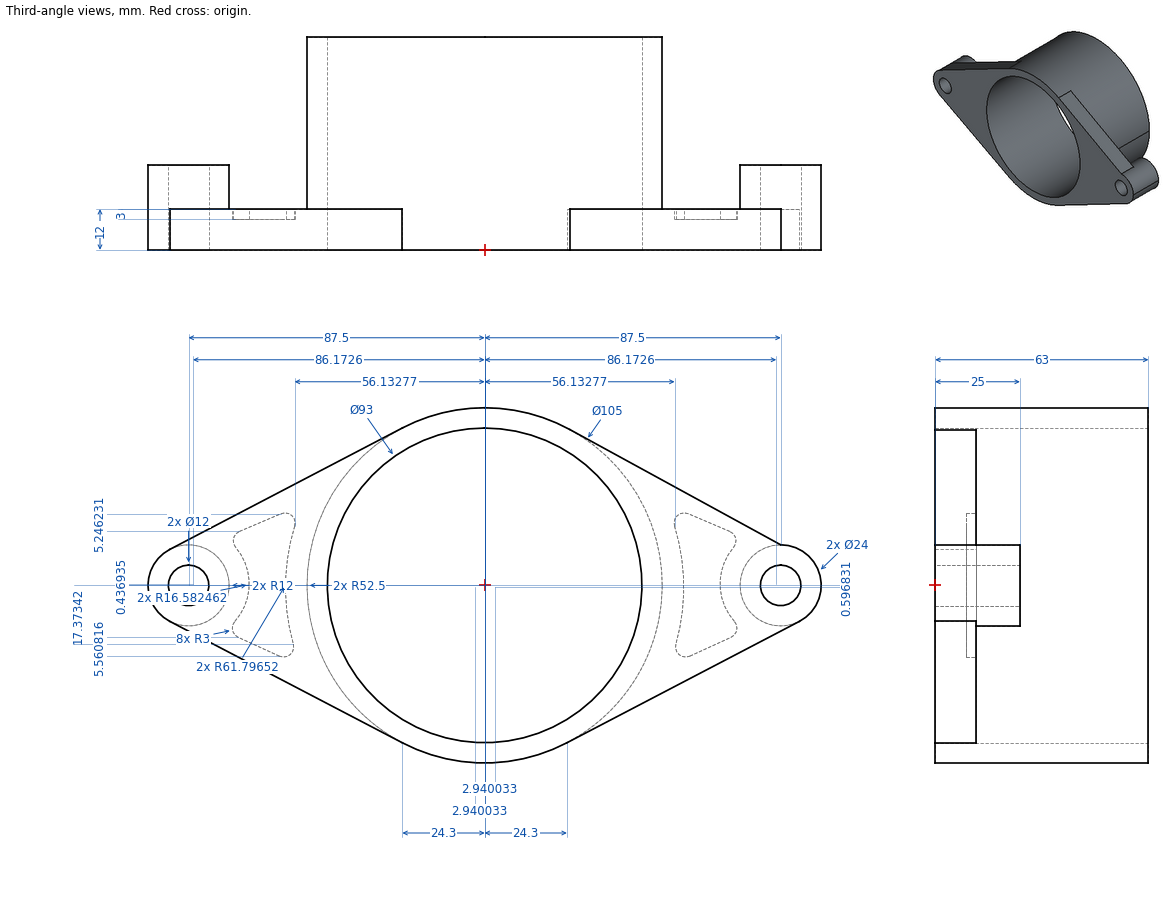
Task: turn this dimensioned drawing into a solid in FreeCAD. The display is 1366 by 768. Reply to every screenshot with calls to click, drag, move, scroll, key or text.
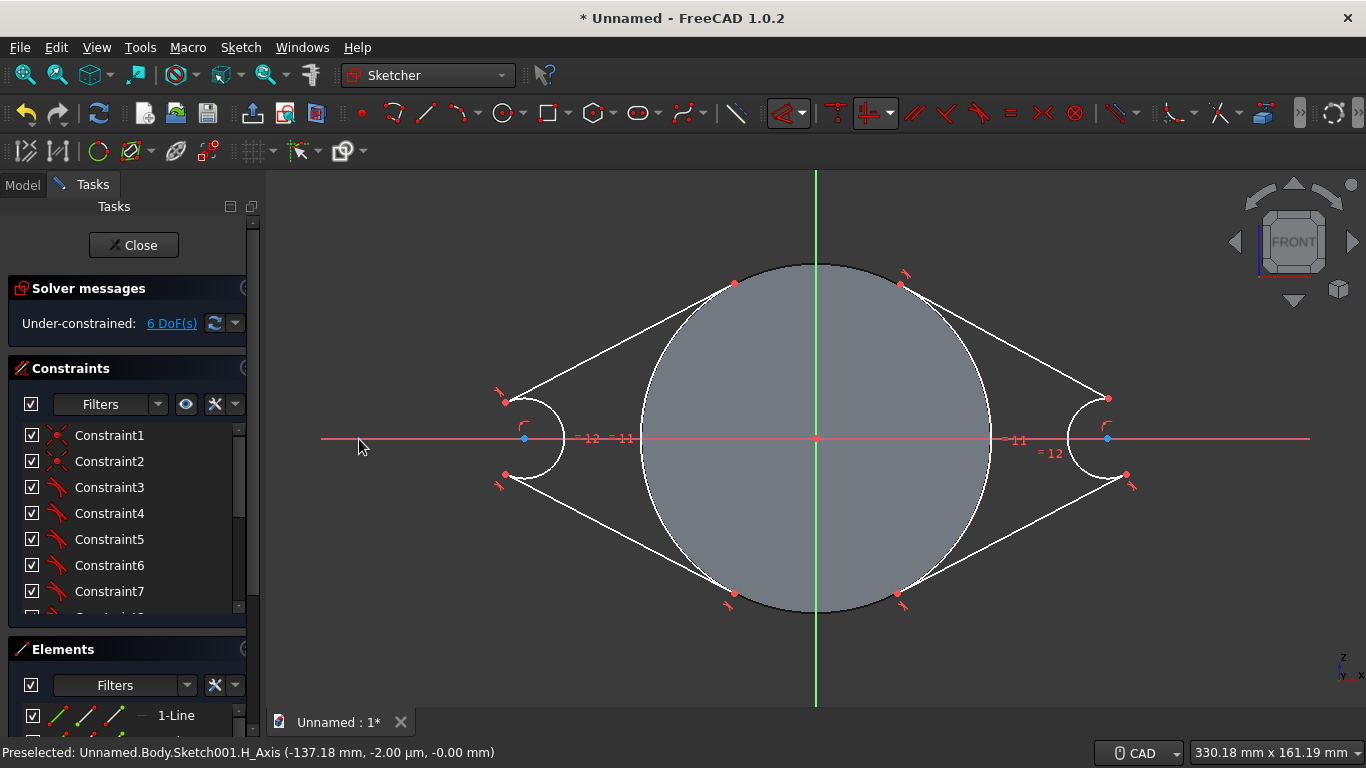
key(d)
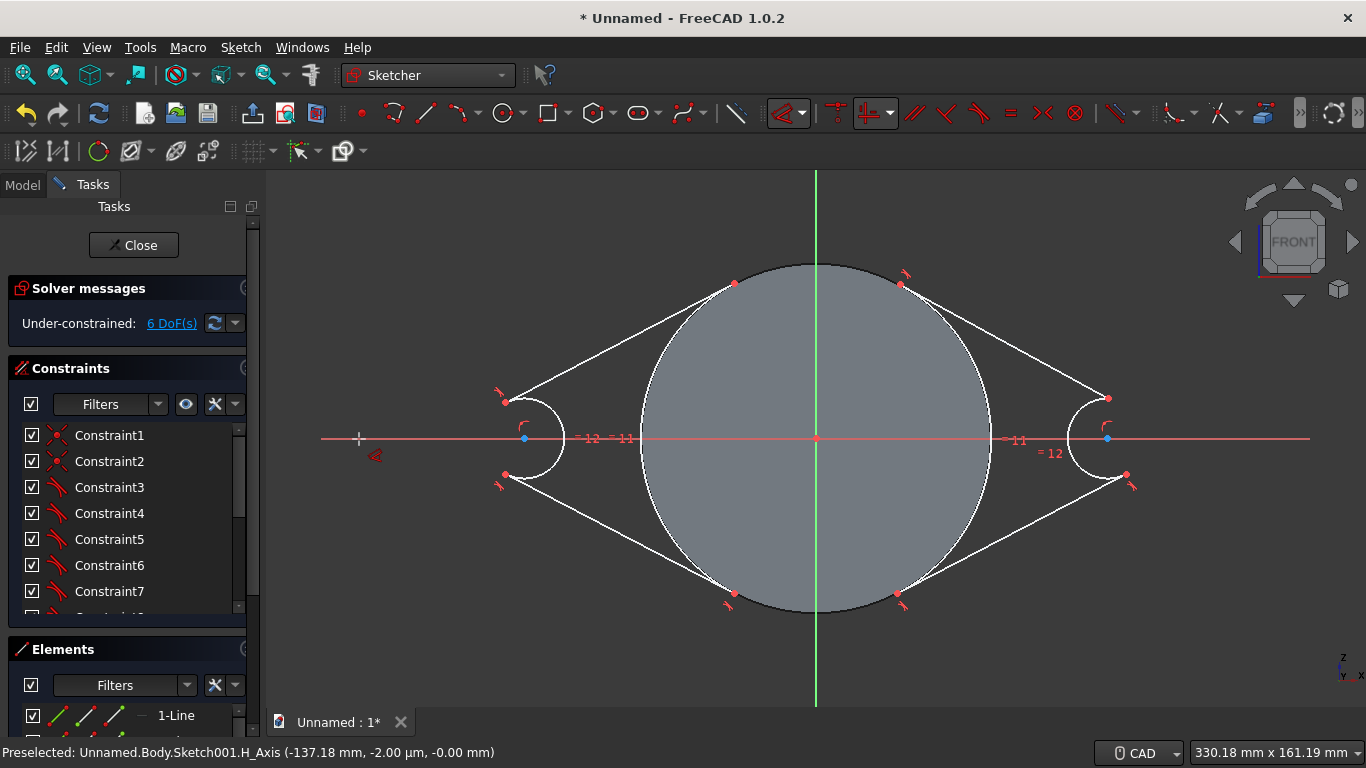
click(552, 468)
click(574, 491)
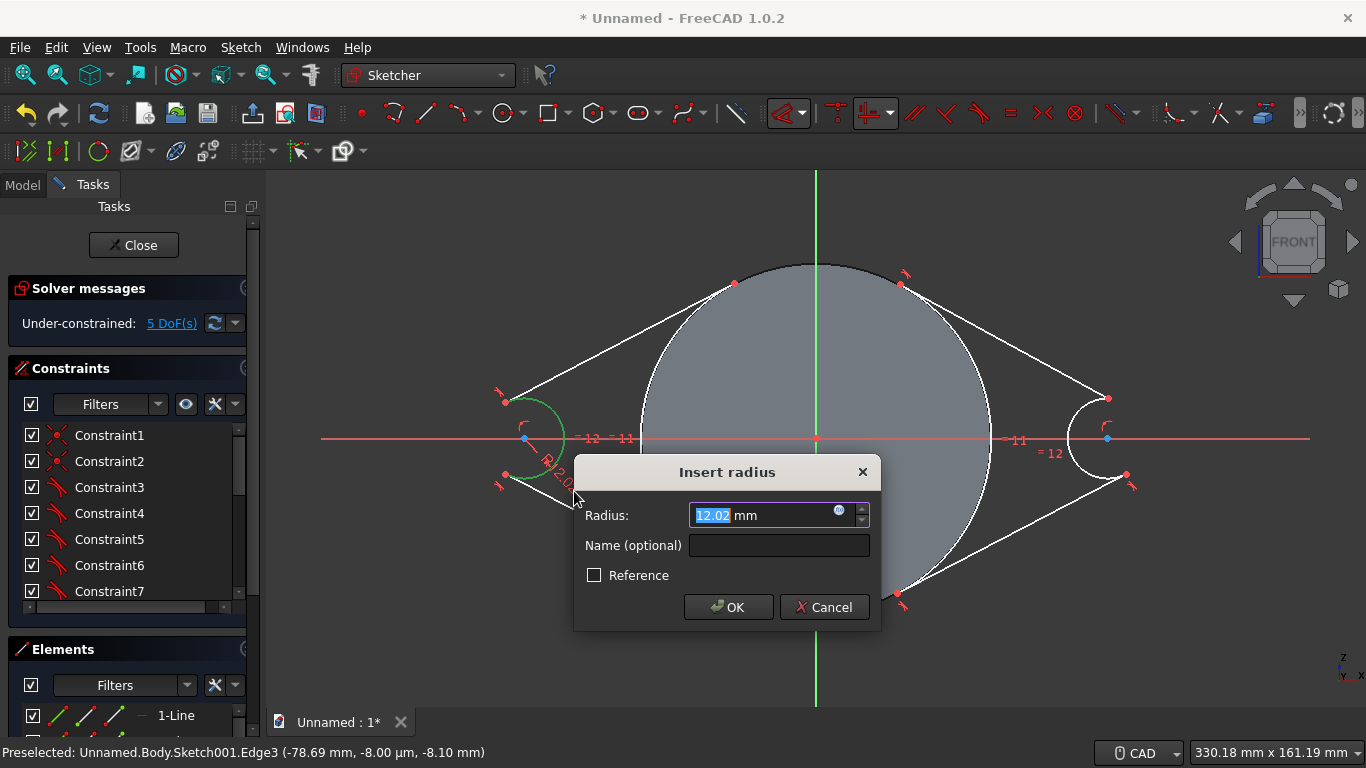
text(12)
key(Return)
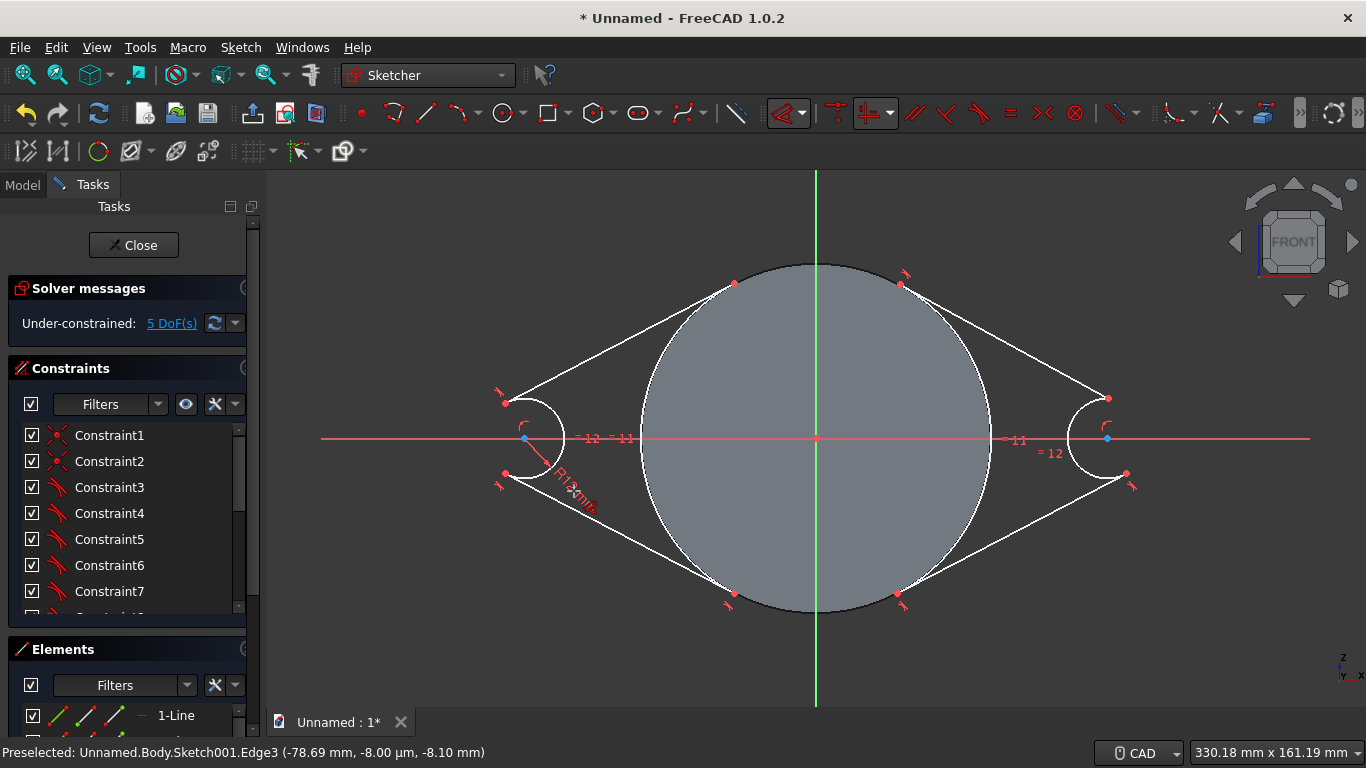
click(657, 365)
click(693, 272)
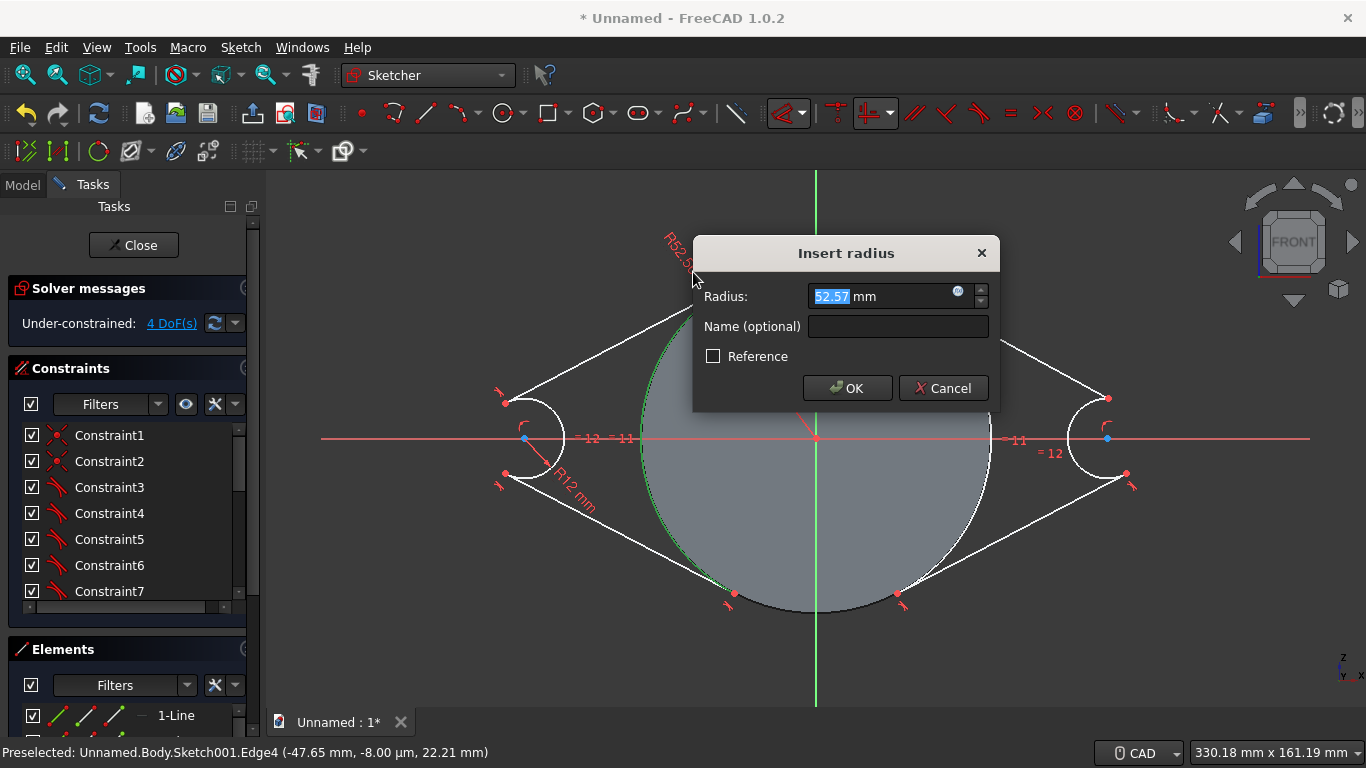
text(52.5)
key(Return)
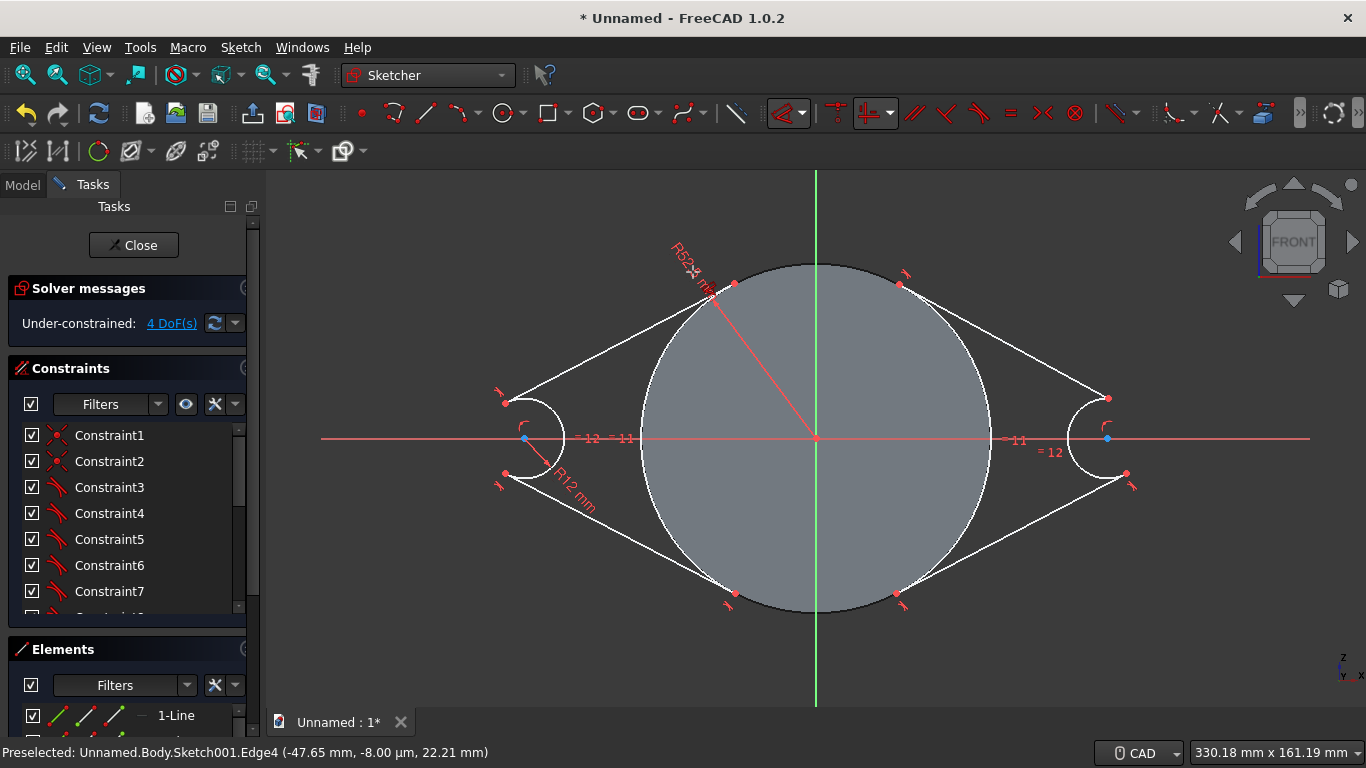
click(735, 594)
click(776, 628)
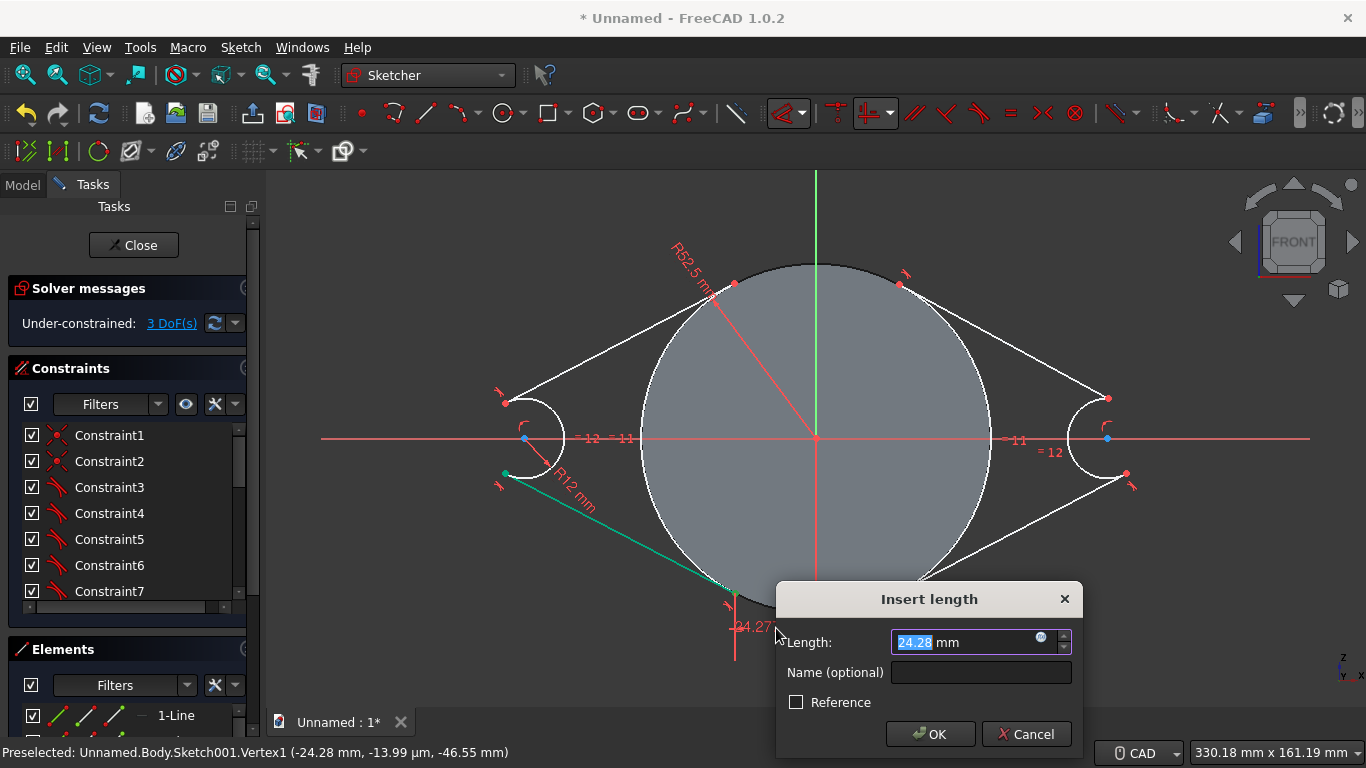
text(24.3)
key(Return)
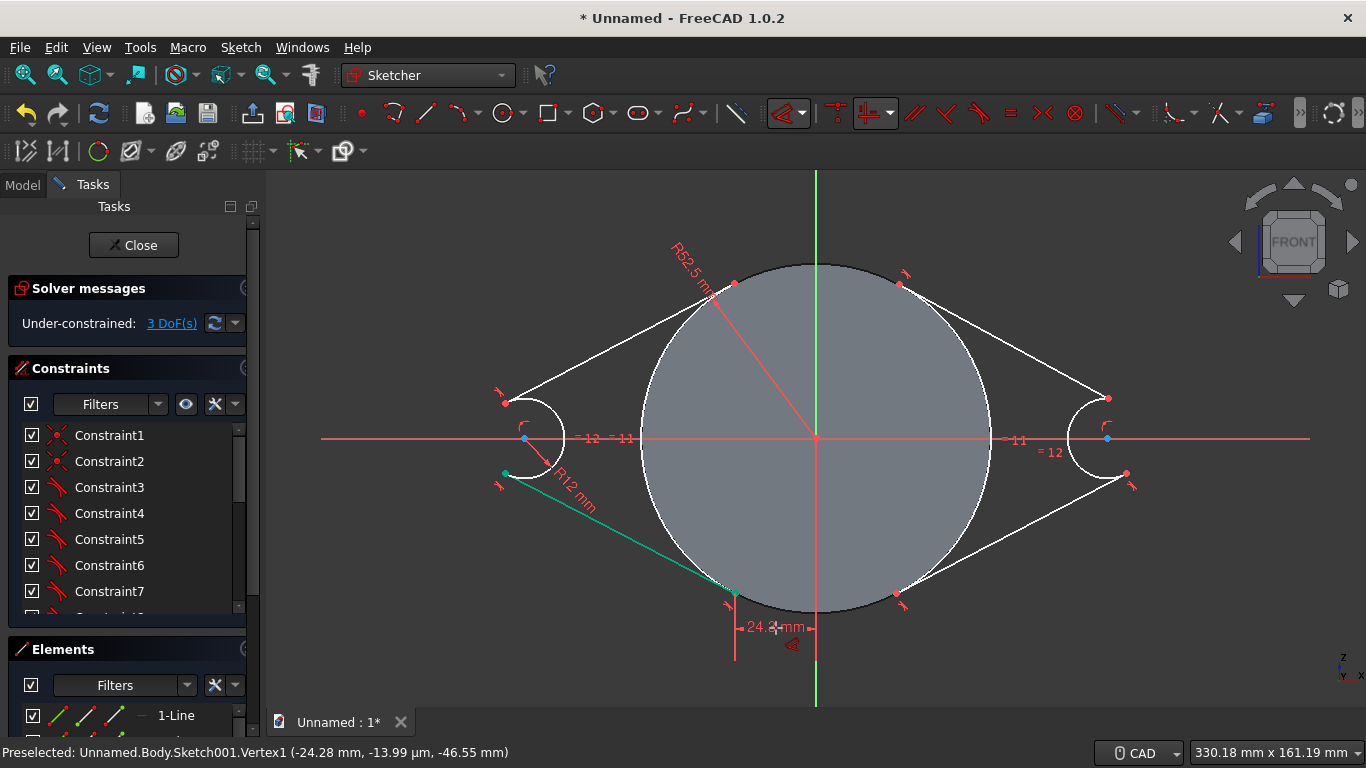
click(735, 283)
click(775, 249)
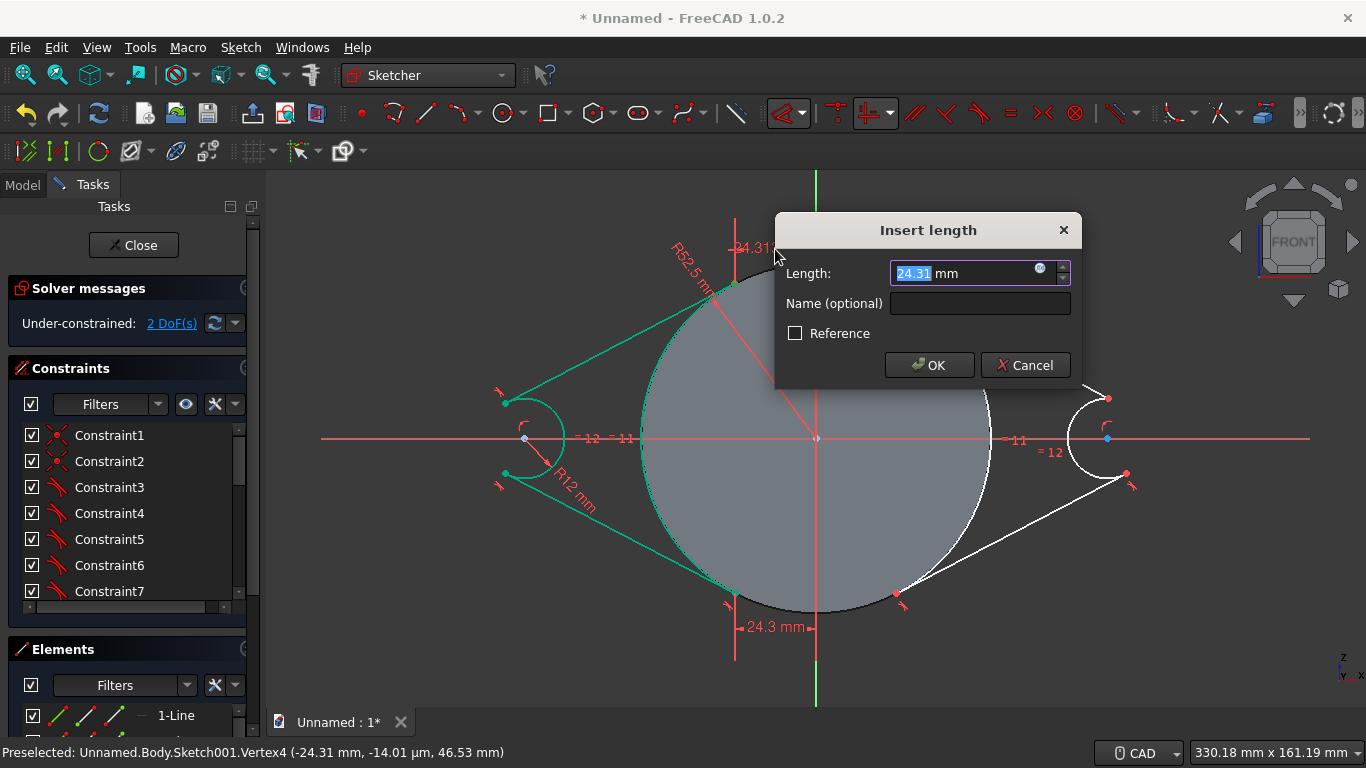
text(24.3)
key(Return)